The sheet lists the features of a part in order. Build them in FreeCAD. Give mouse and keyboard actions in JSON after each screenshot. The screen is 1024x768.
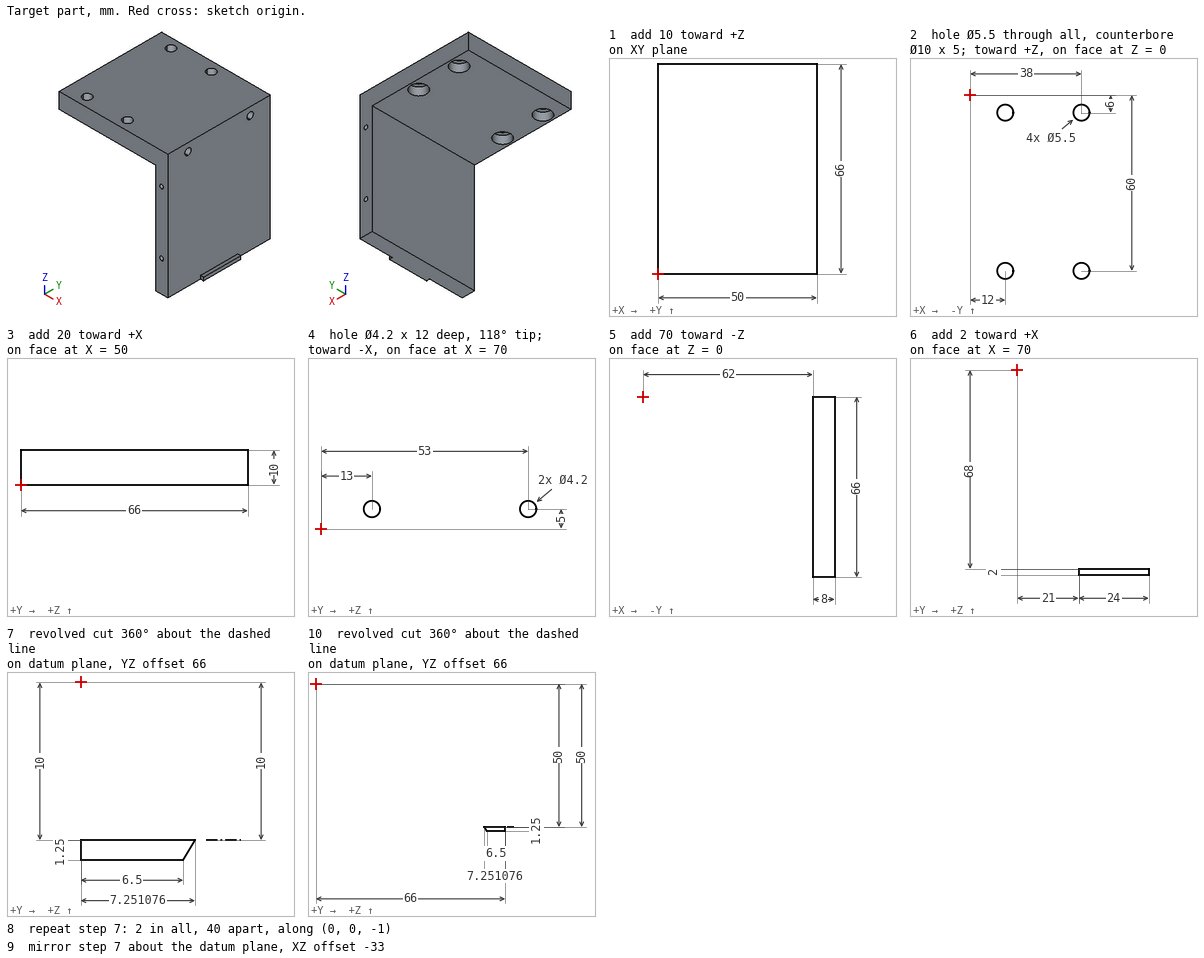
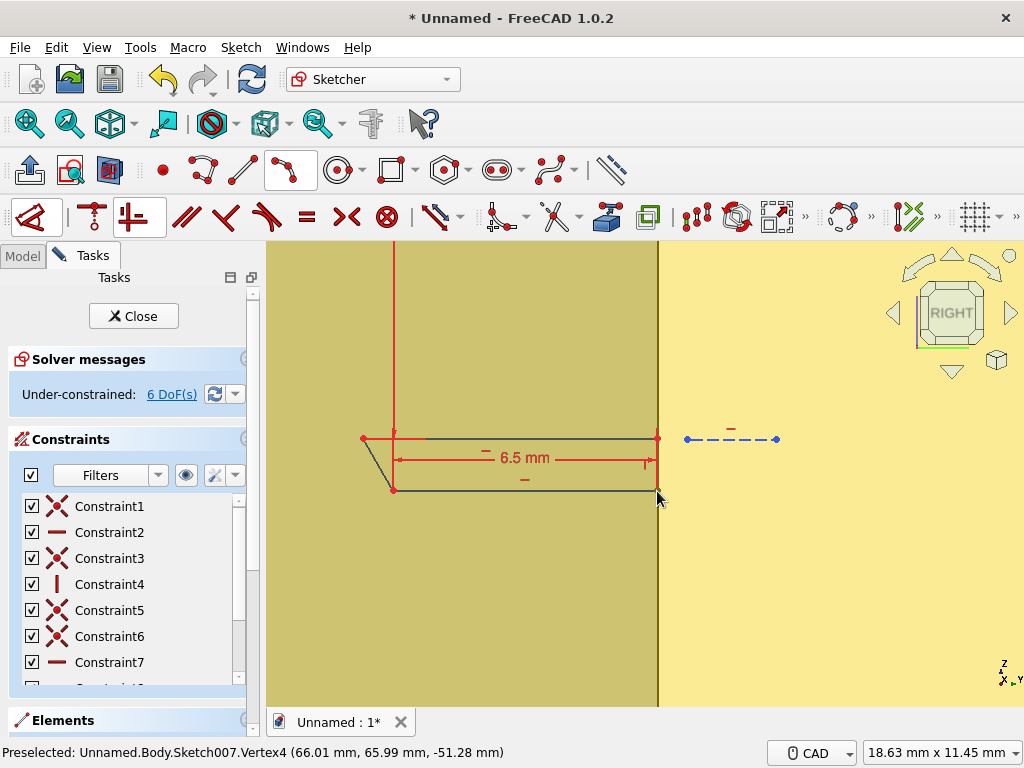
{"action": "key", "text": "l"}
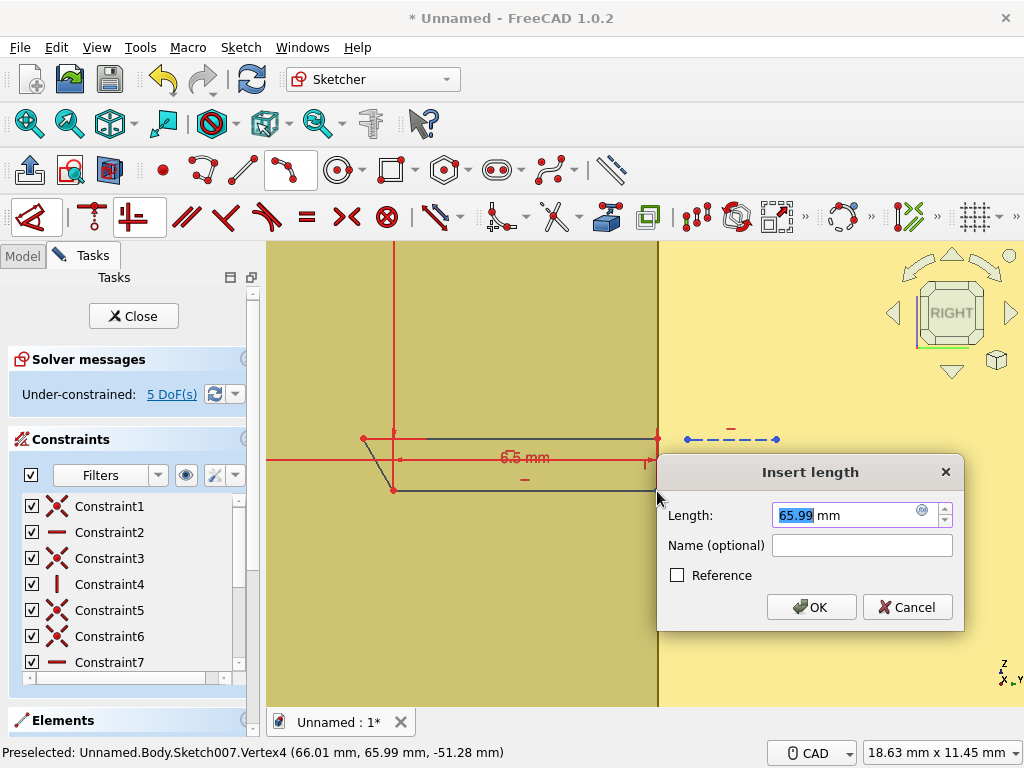
{"action": "type", "text": "66"}
{"action": "key", "text": "Return"}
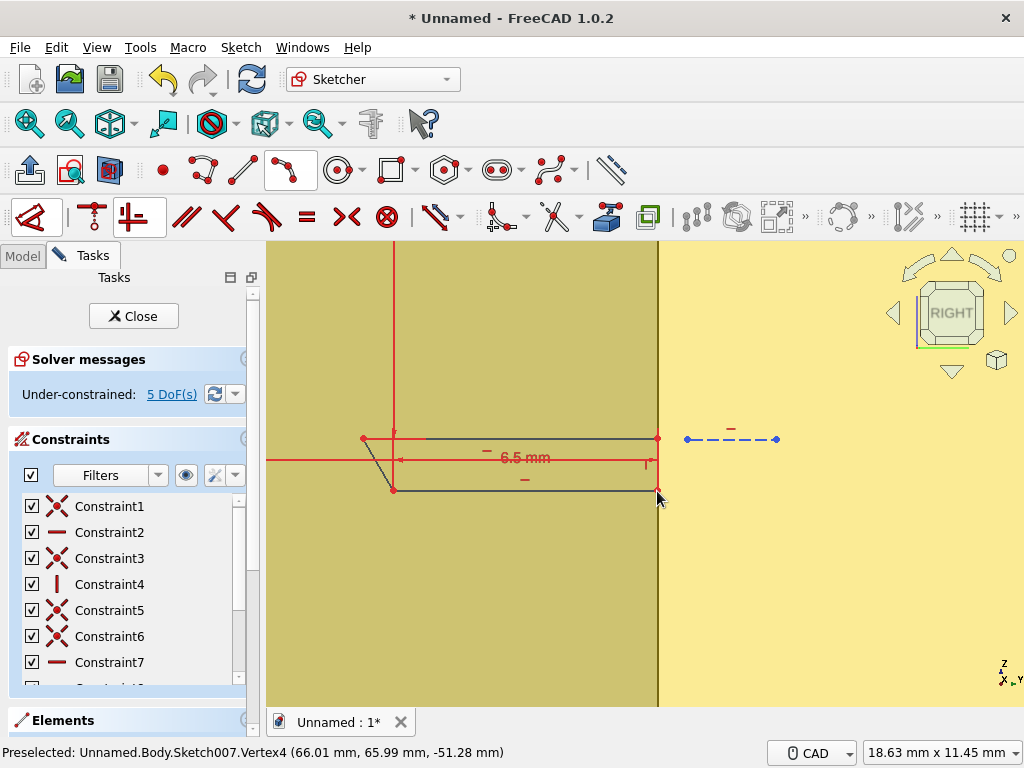
{"action": "left_click", "coordinate": [687, 440]}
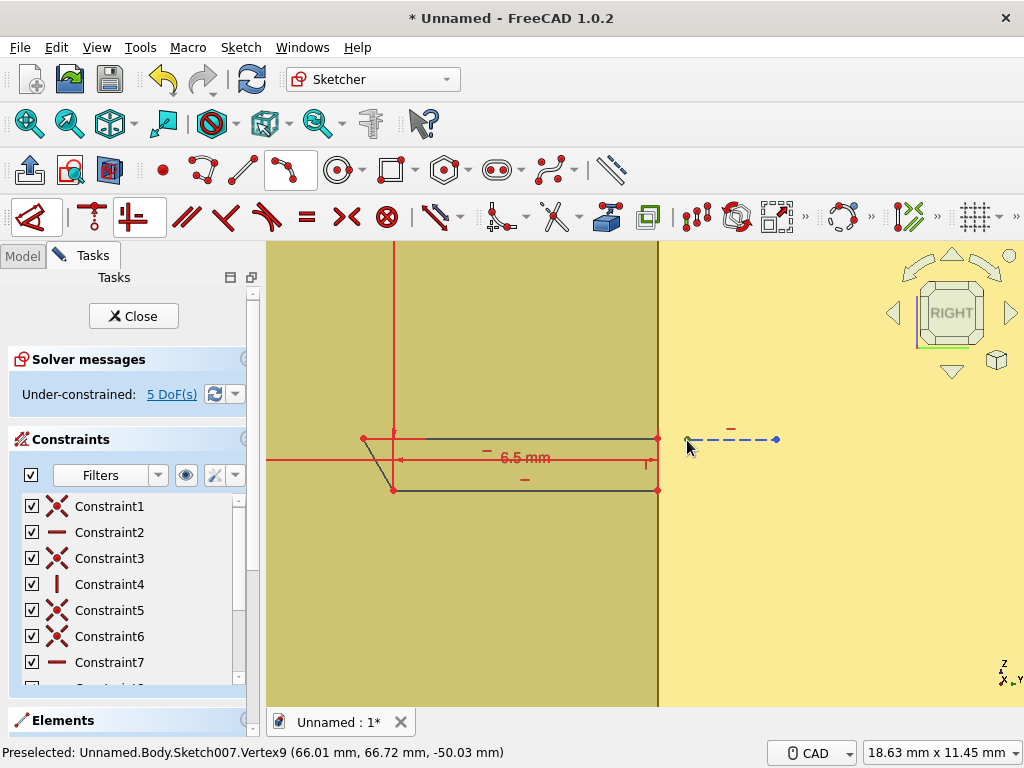
{"action": "left_click", "coordinate": [56, 218]}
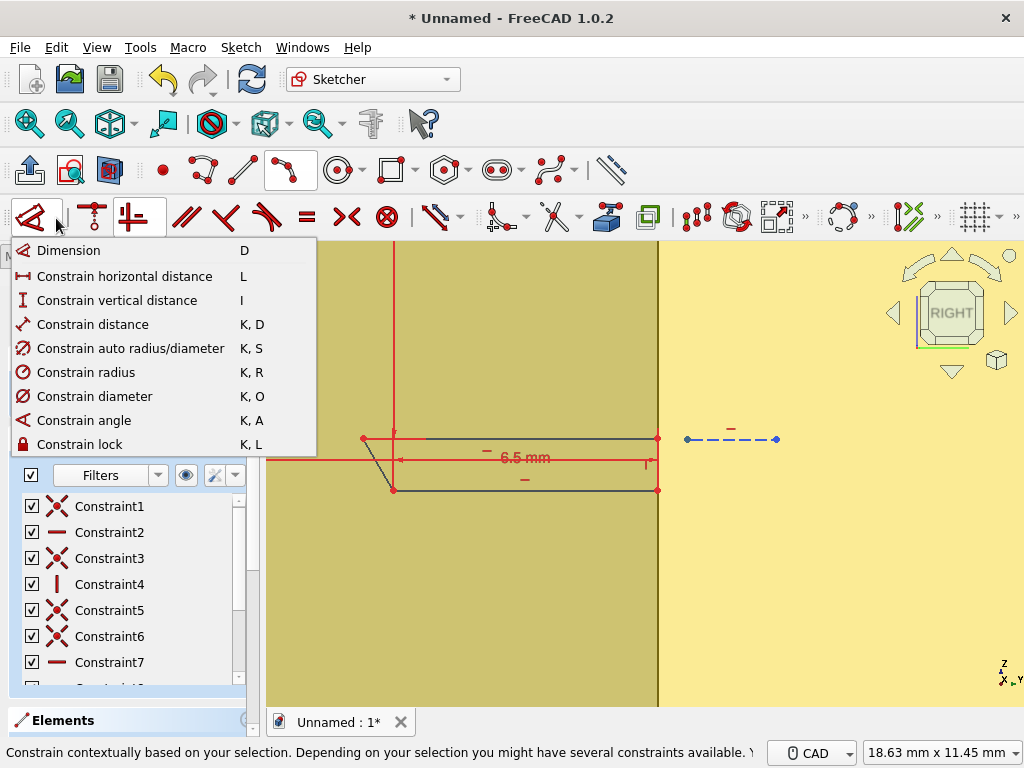
{"action": "left_click", "coordinate": [164, 300]}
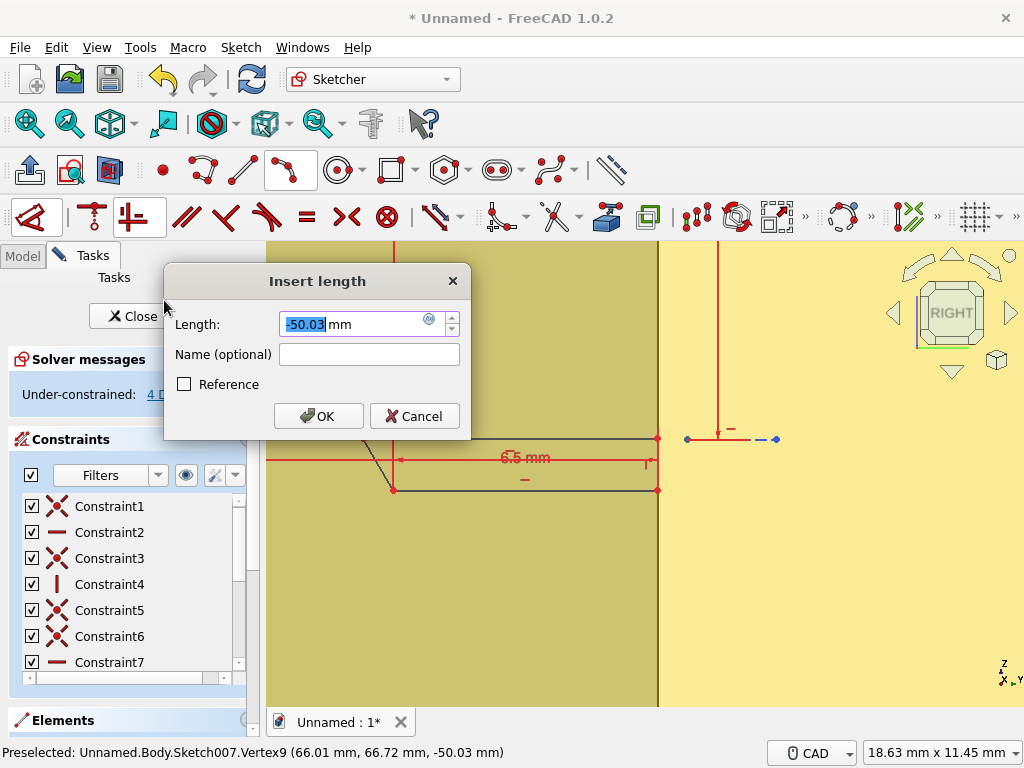
{"action": "type", "text": "-50"}
{"action": "key", "text": "Return"}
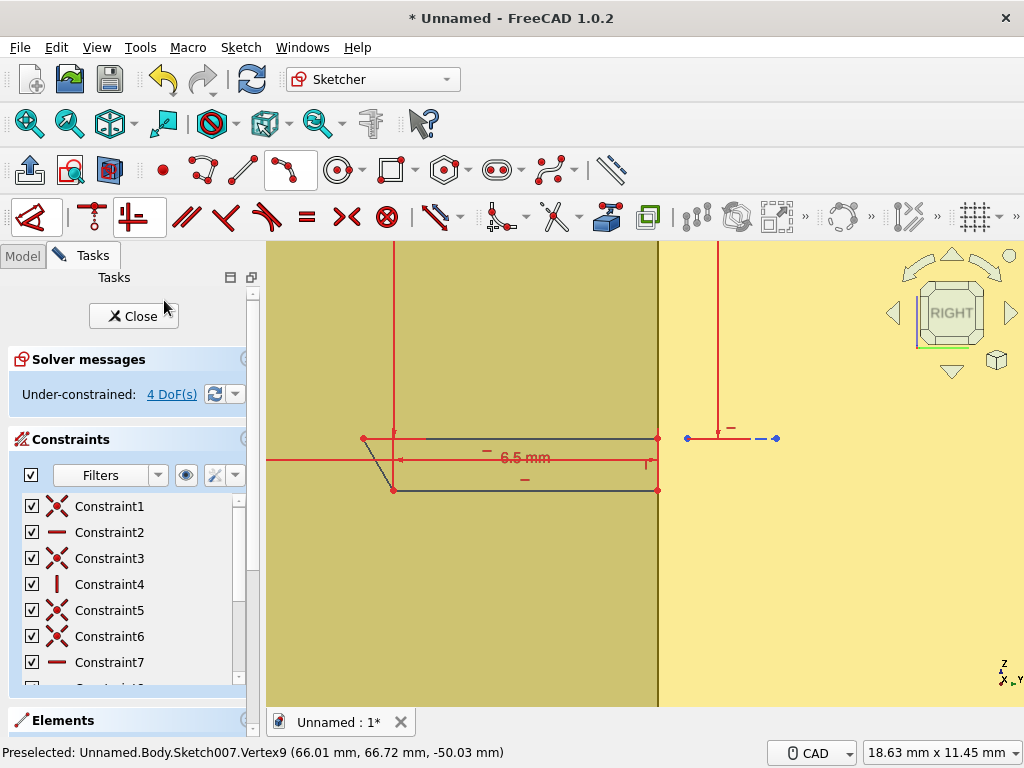
{"action": "left_click", "coordinate": [658, 475]}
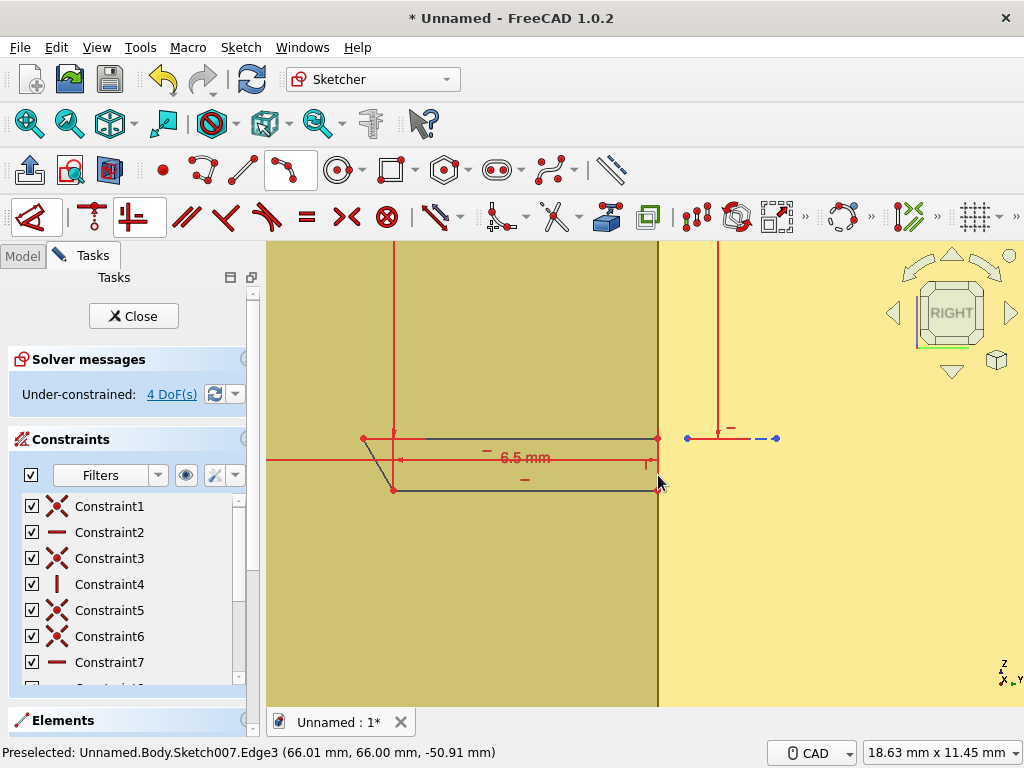
{"action": "key", "text": "i"}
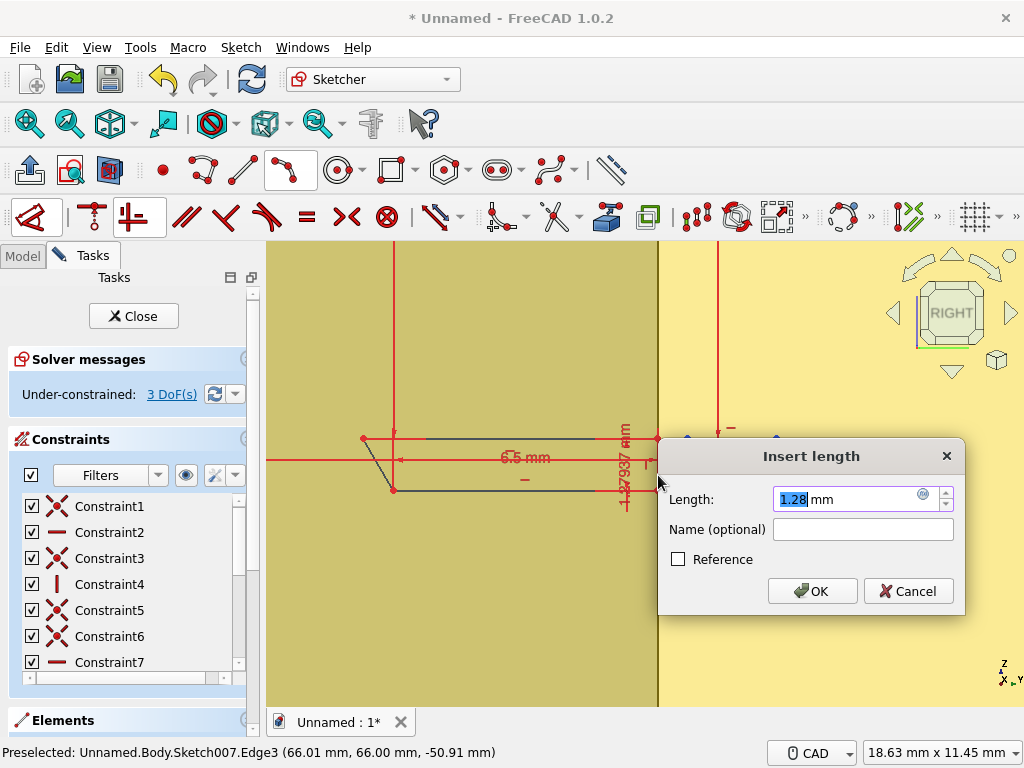
{"action": "type", "text": "1.25"}
{"action": "key", "text": "Return"}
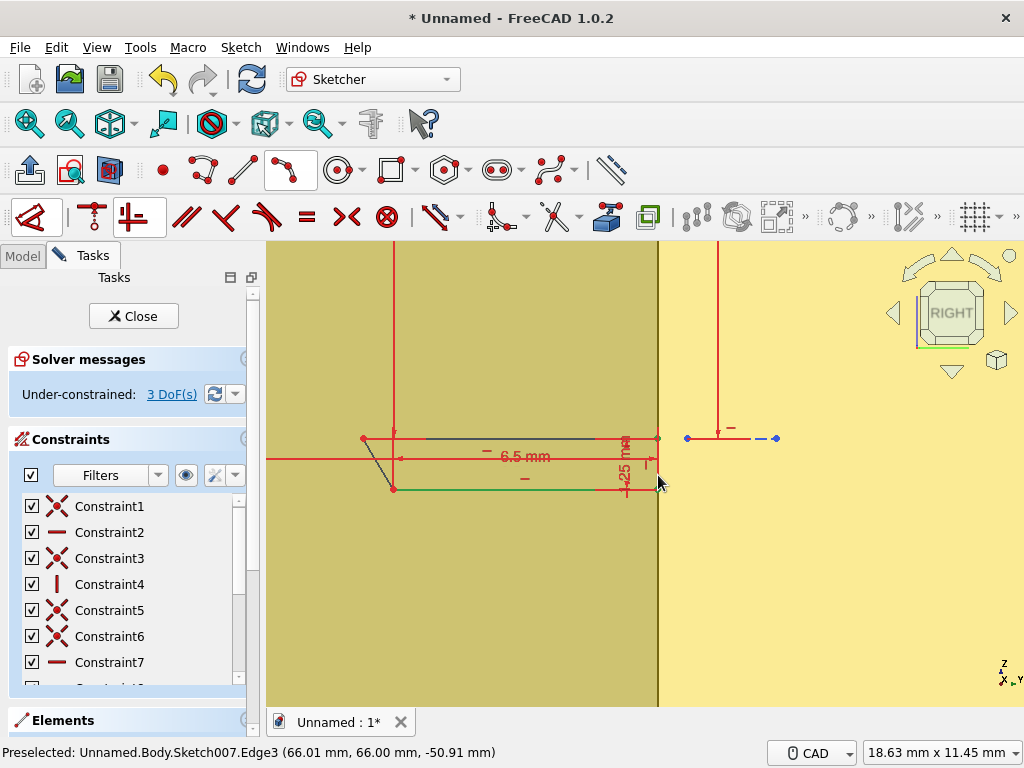
{"action": "left_click", "coordinate": [569, 439]}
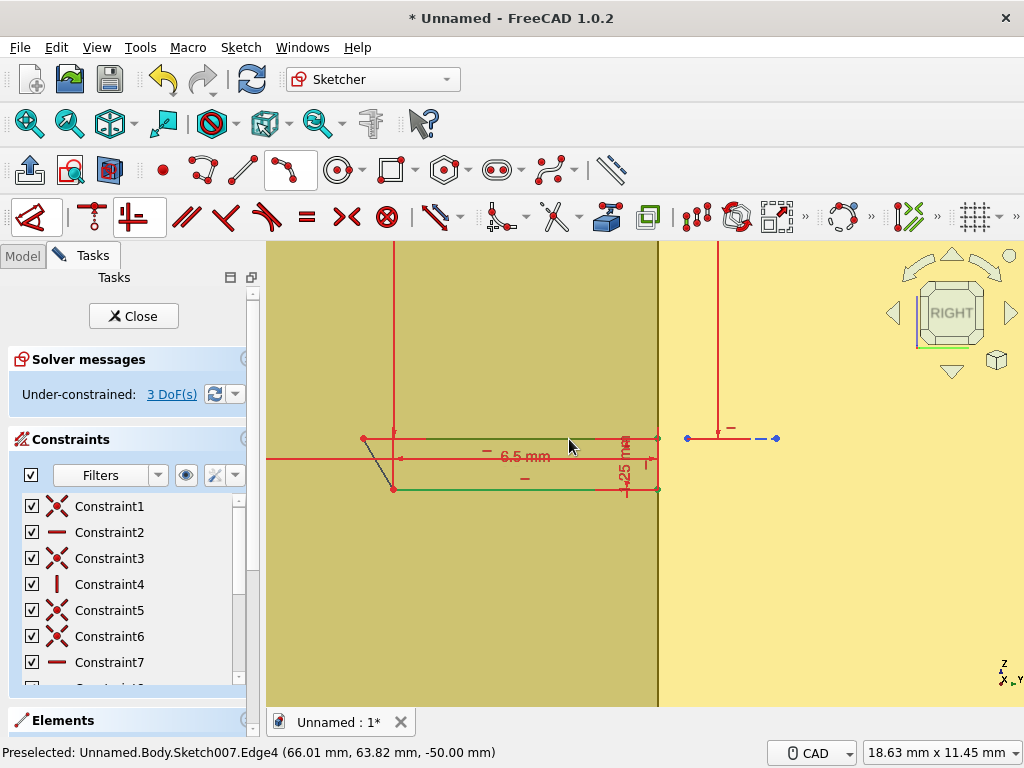
{"action": "key", "text": "l"}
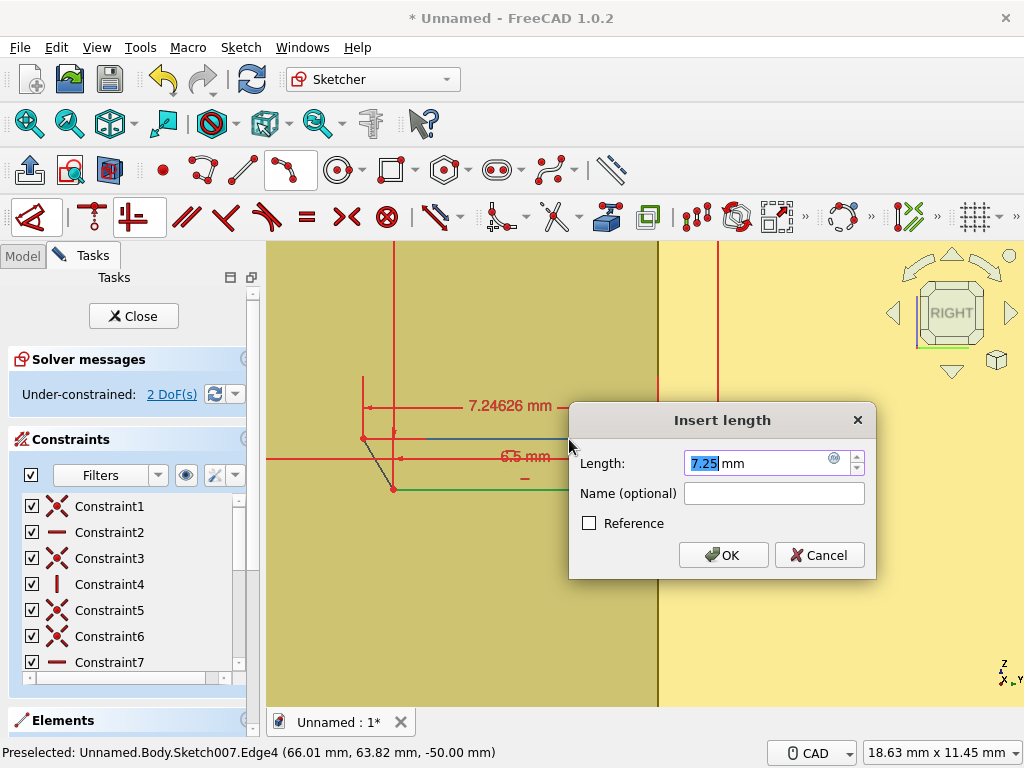
{"action": "type", "text": "7.251076"}
{"action": "key", "text": "Return"}